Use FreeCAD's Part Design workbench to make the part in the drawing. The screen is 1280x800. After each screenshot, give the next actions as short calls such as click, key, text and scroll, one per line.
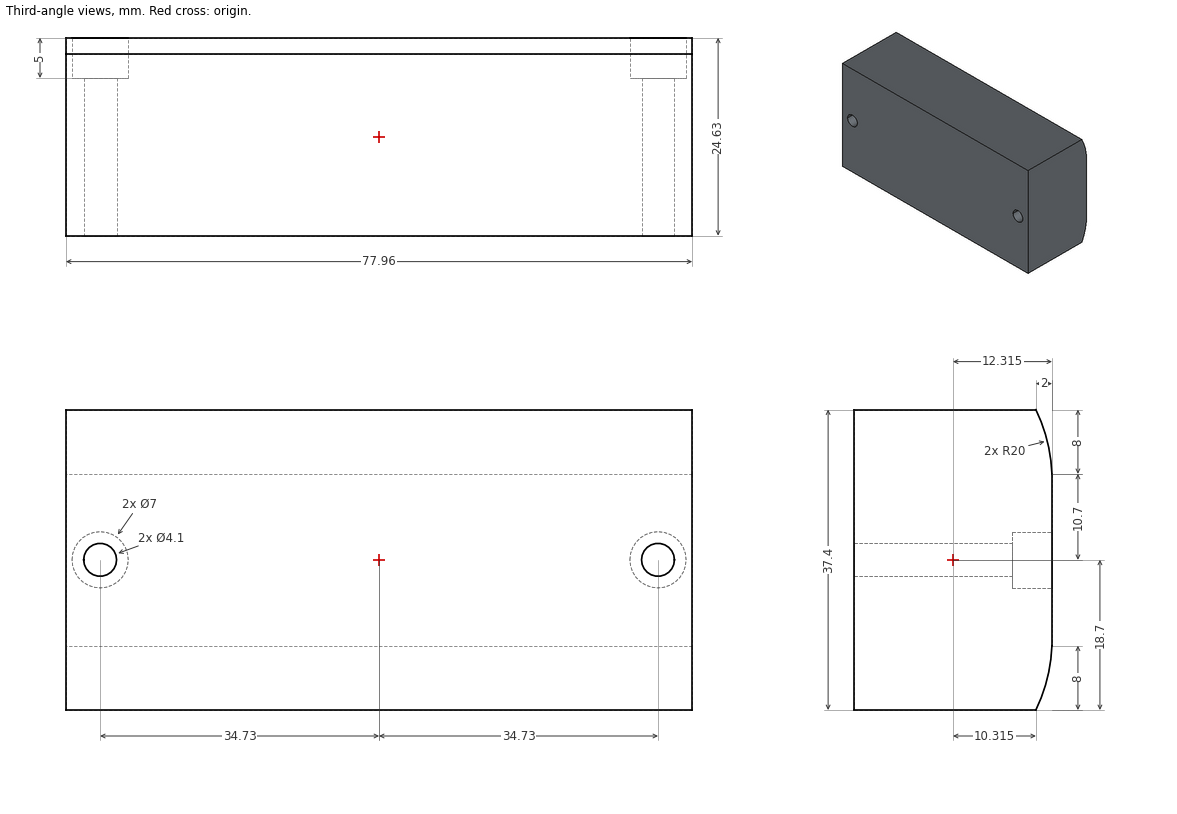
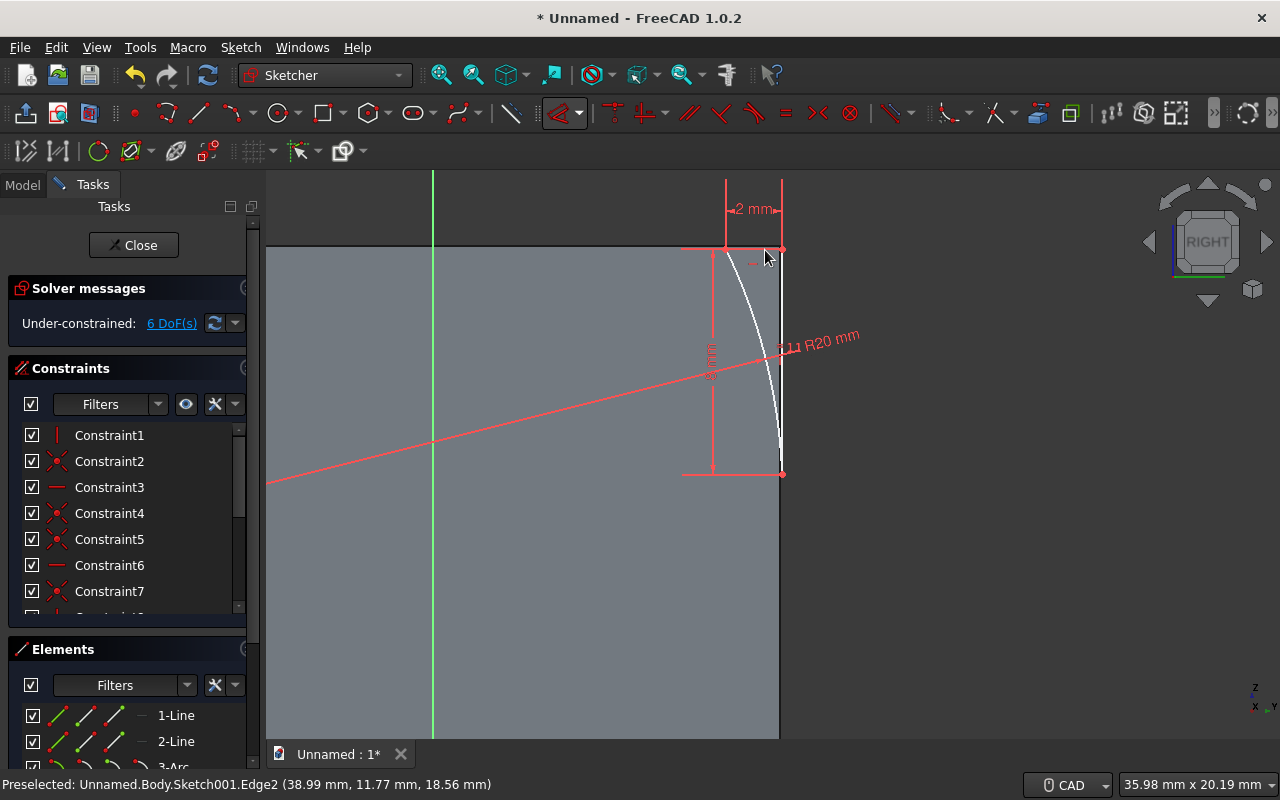
scroll(761, 269, down, 5)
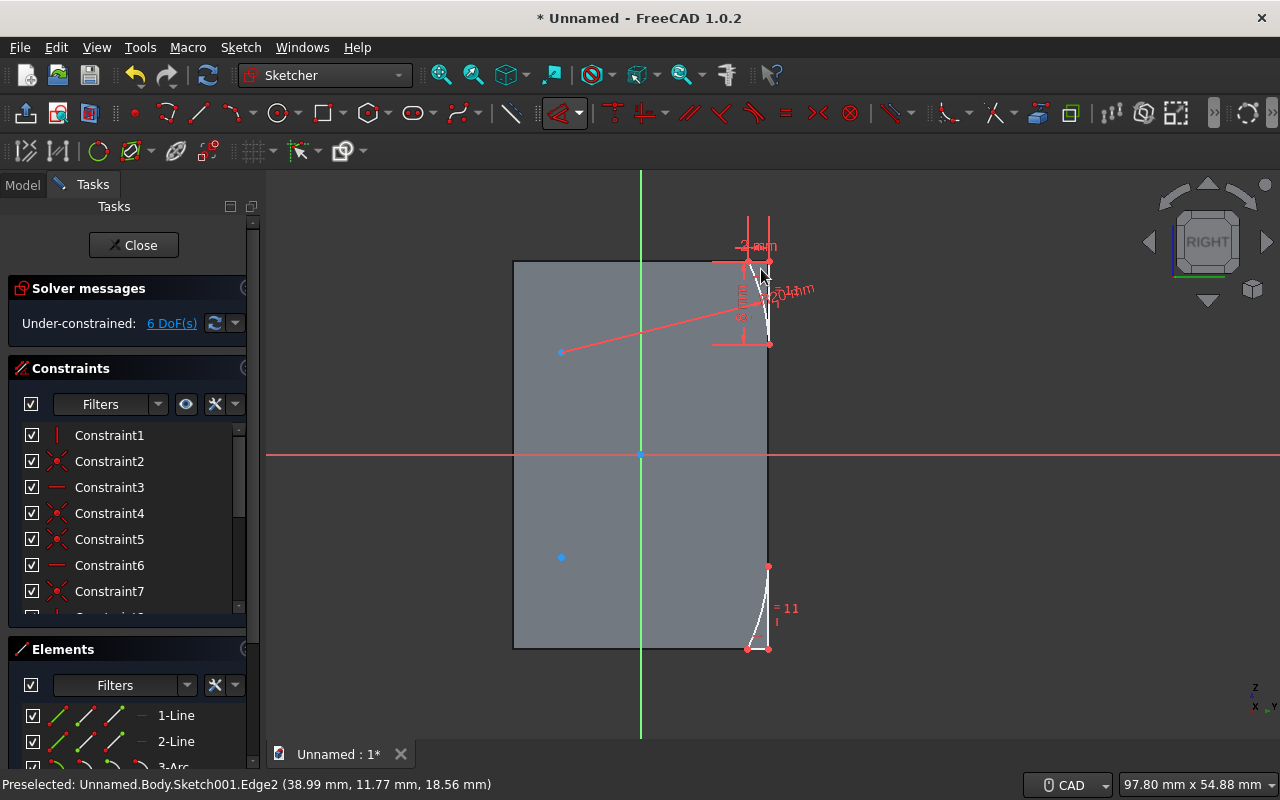
scroll(754, 649, up, 5)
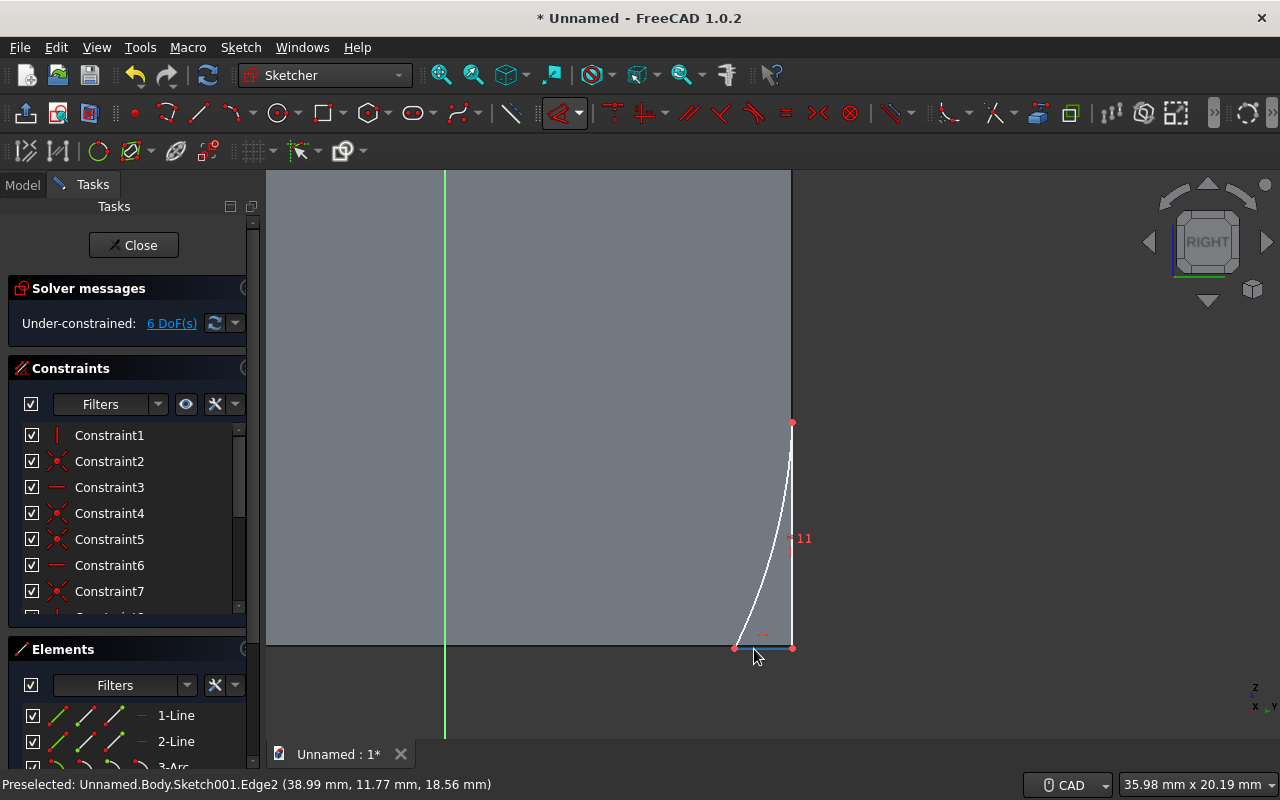
click(752, 648)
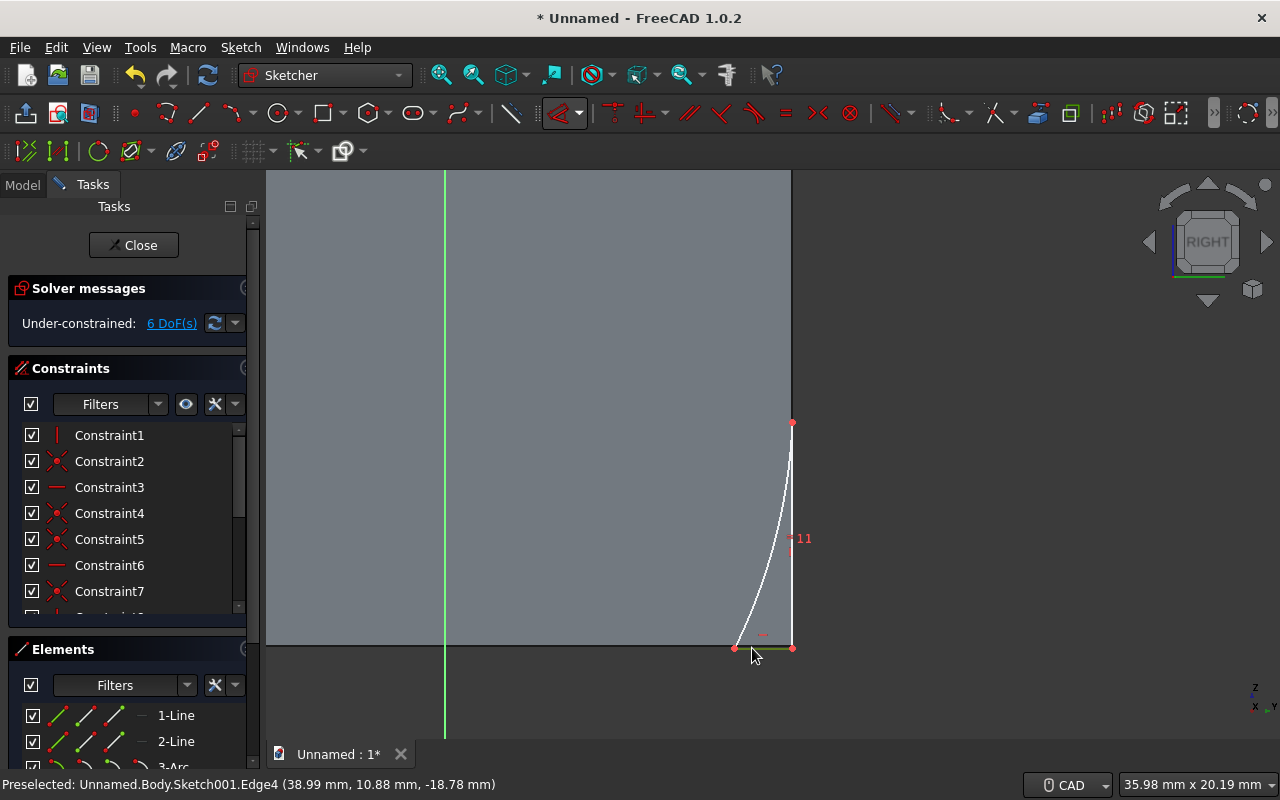
click(582, 114)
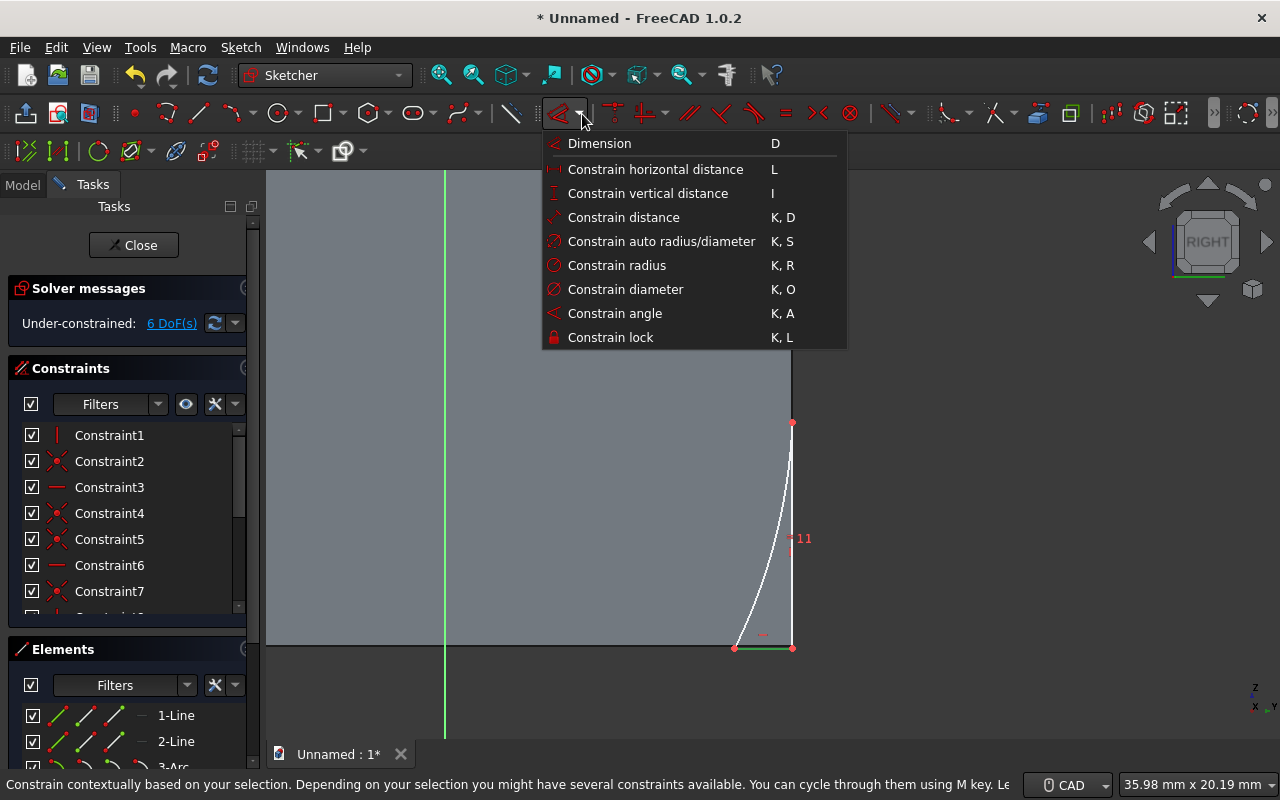
click(695, 169)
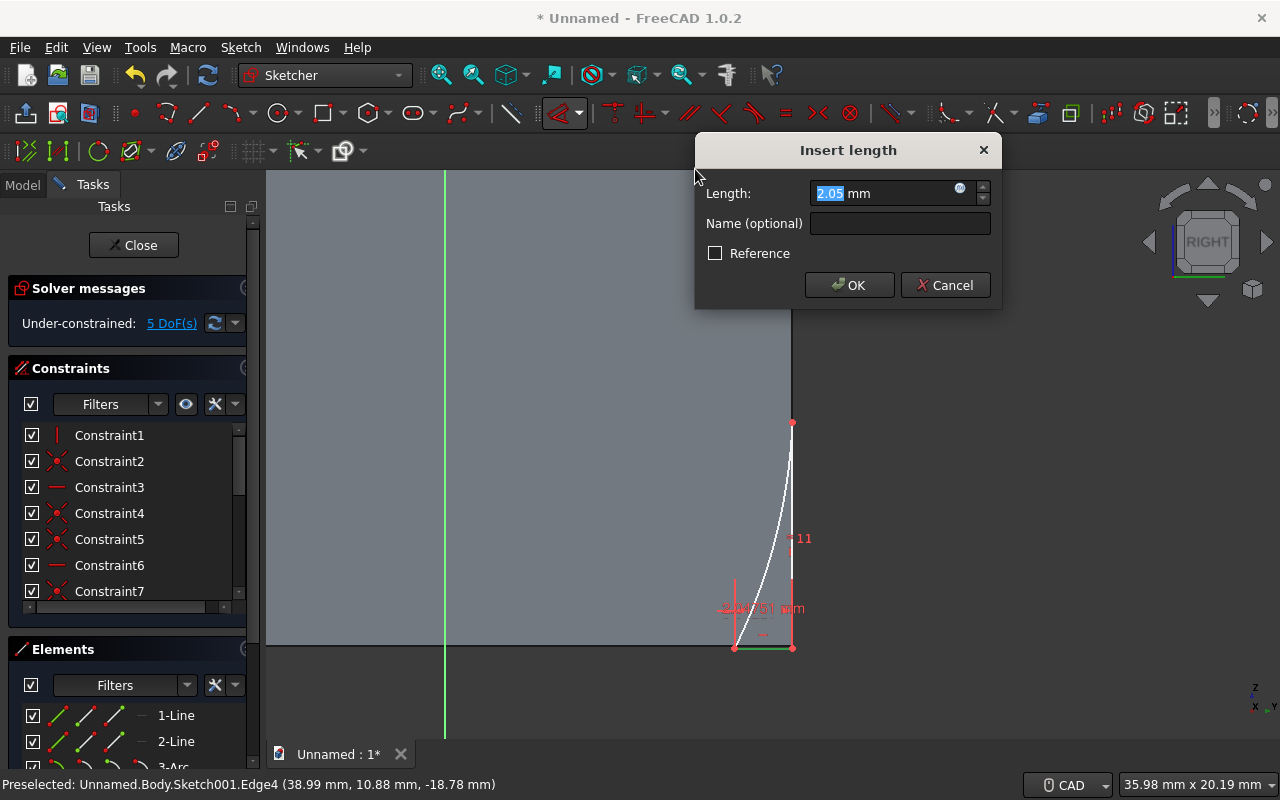
text(2)
key(Return)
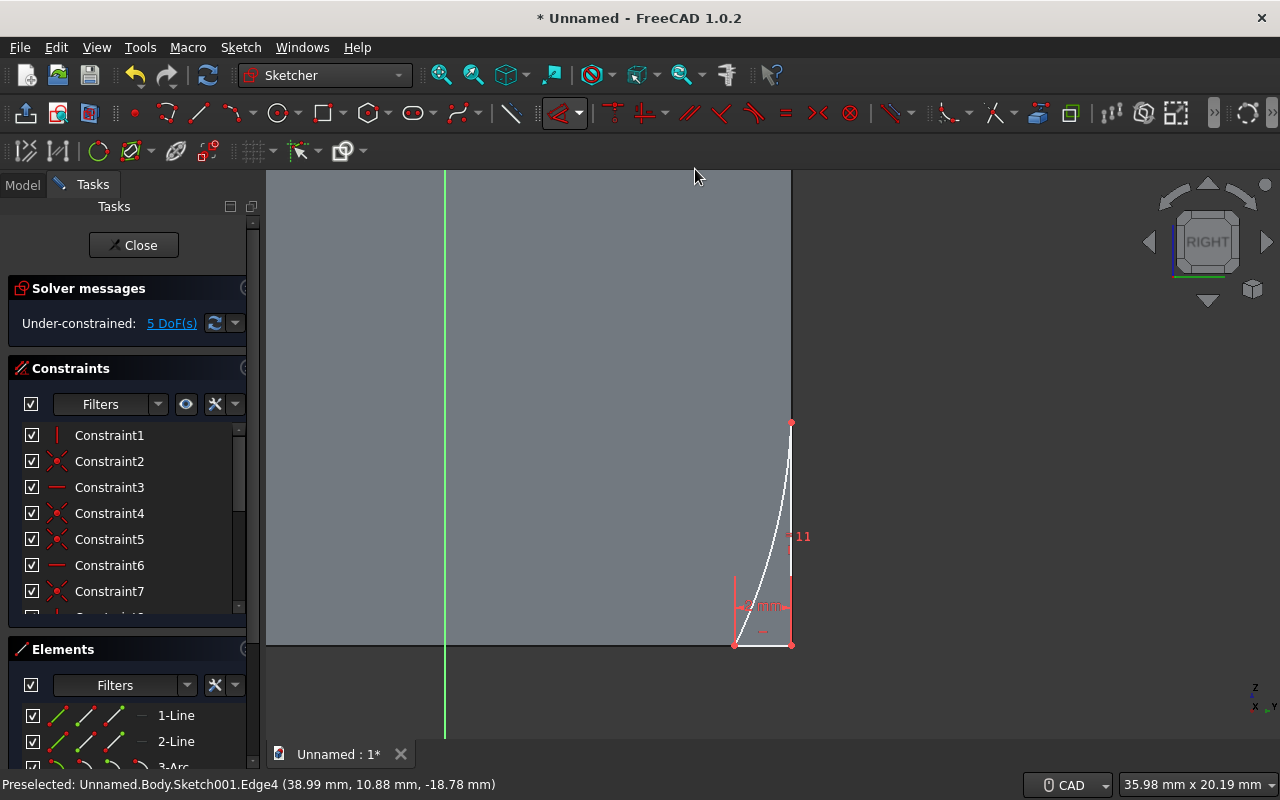
click(791, 579)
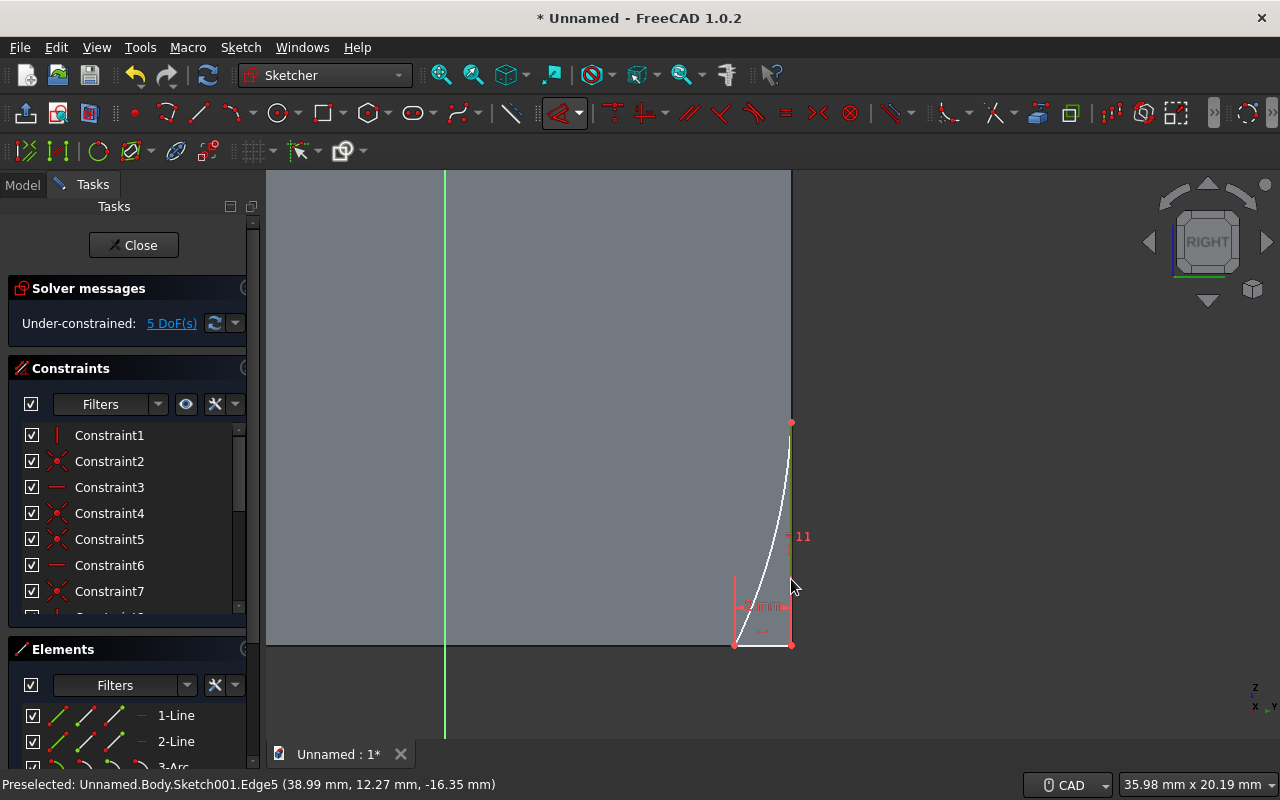
key(i)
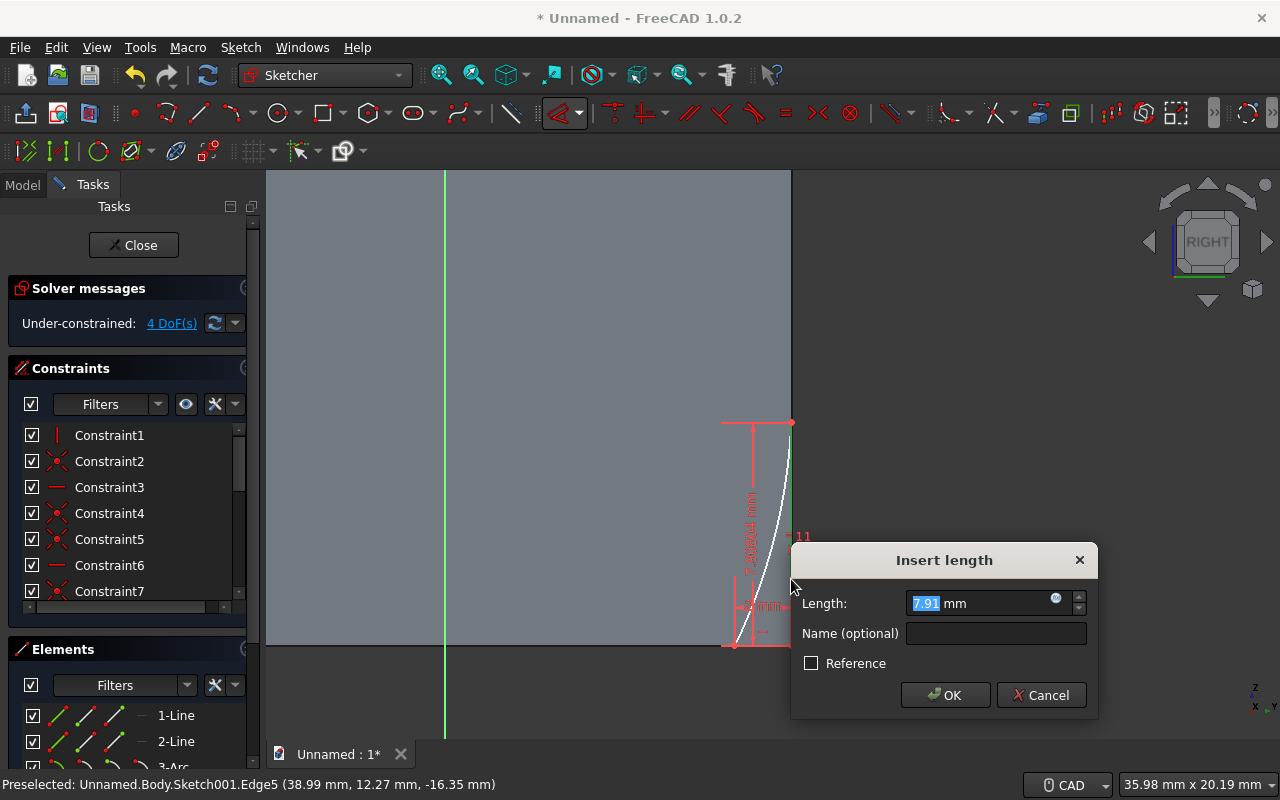
text(8)
key(Return)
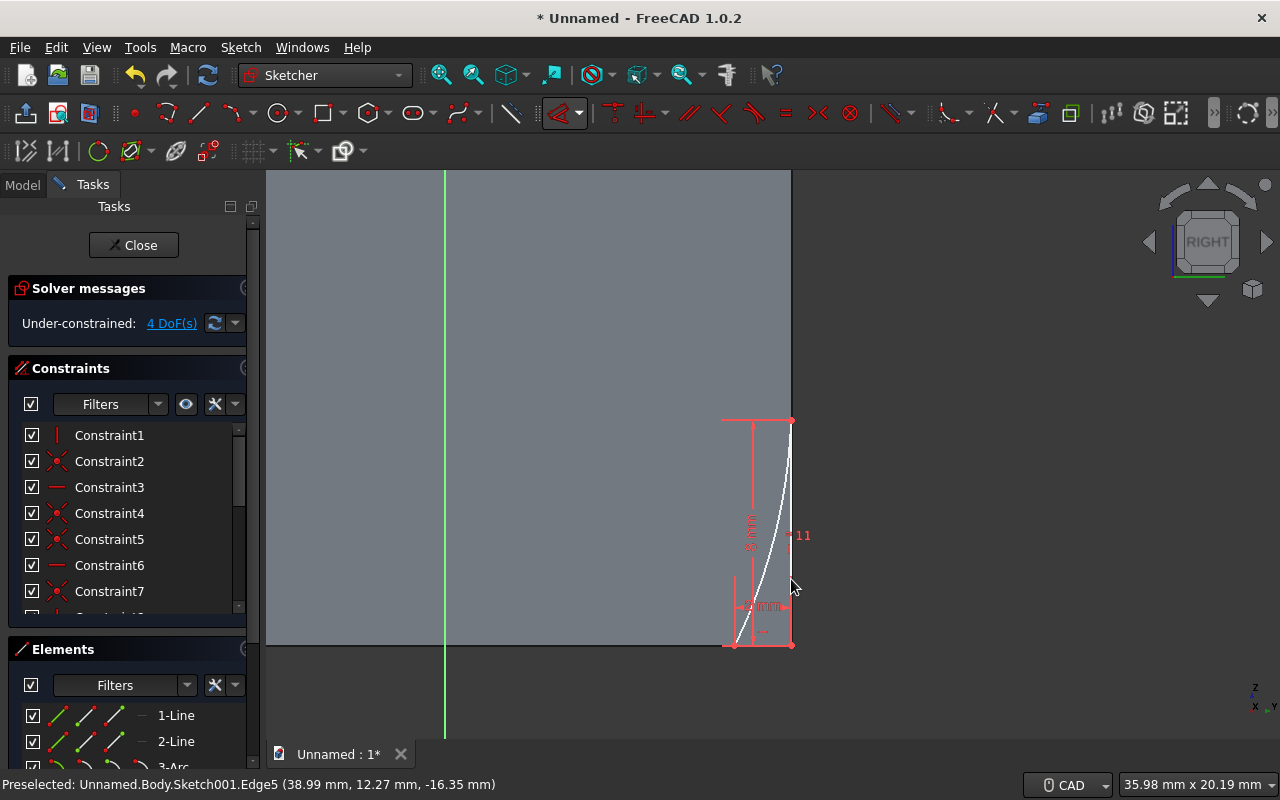
scroll(754, 650, down, 5)